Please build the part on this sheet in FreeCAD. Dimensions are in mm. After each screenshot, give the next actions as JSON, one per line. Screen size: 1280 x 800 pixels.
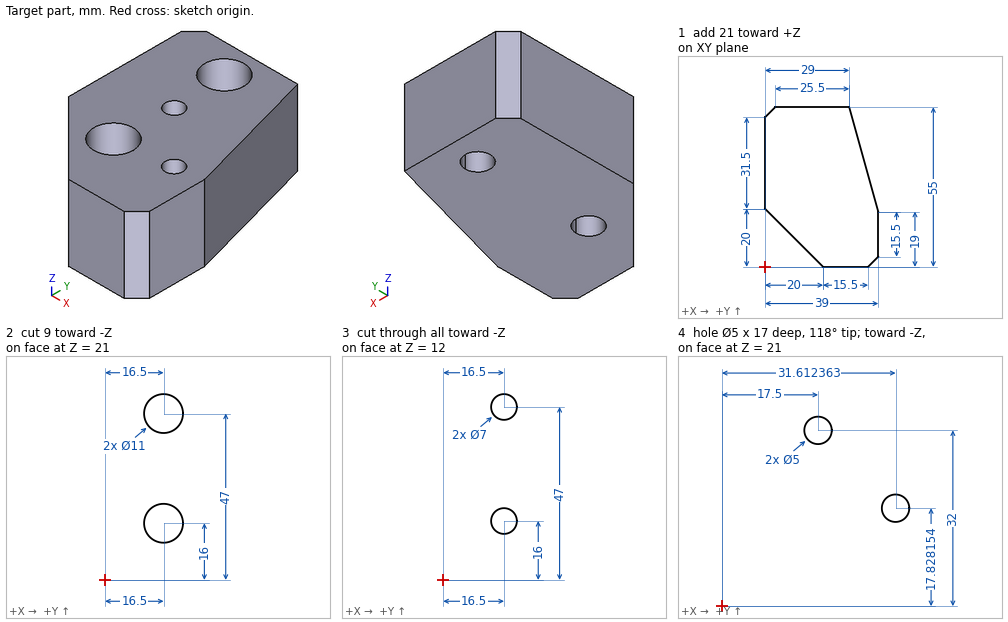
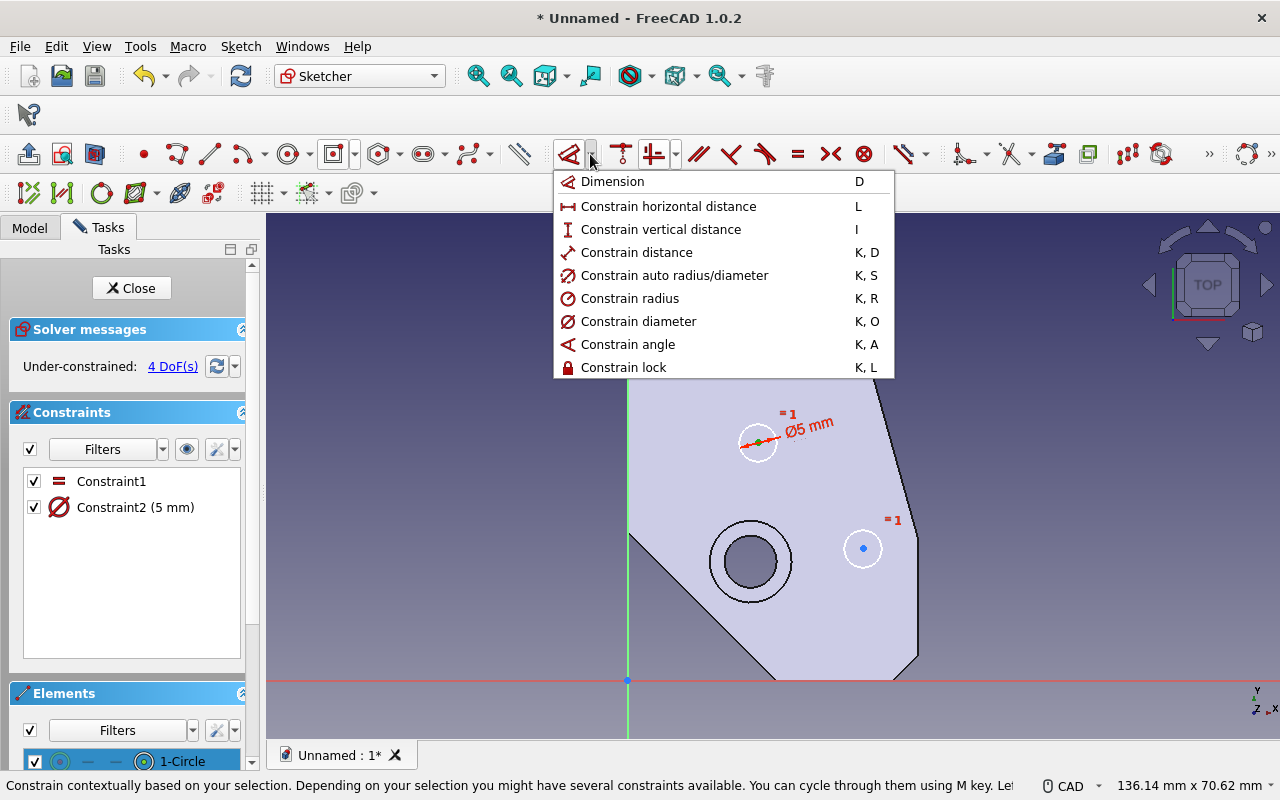
{"action": "left_click", "coordinate": [724, 230]}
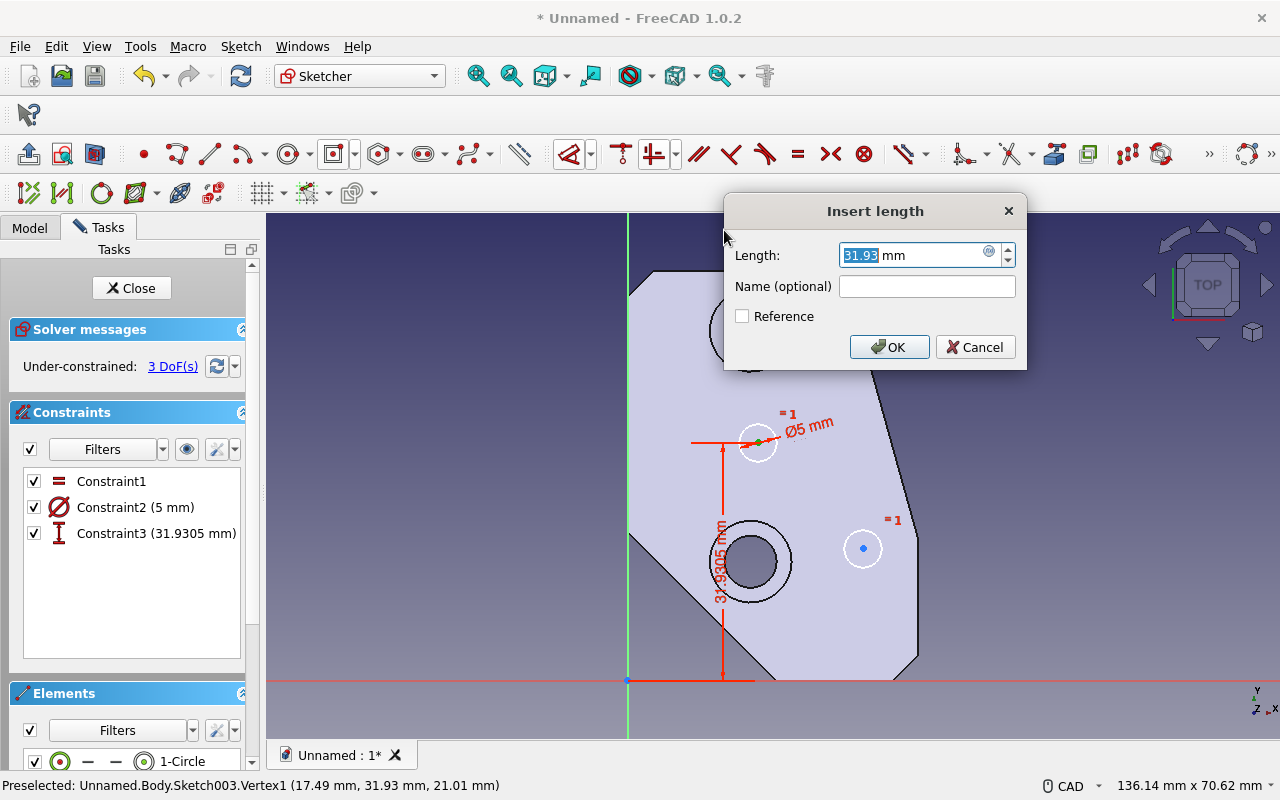
{"action": "type", "text": "32"}
{"action": "key", "text": "Return"}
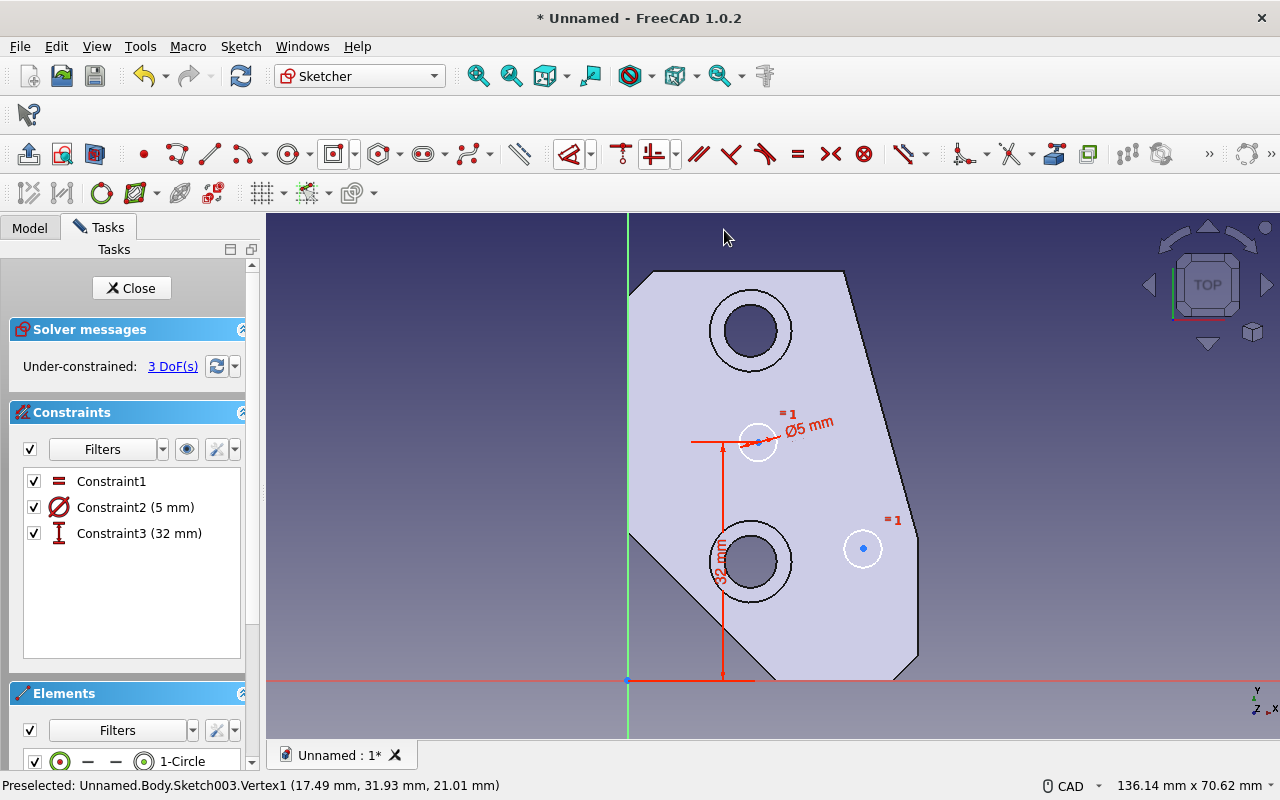
{"action": "left_click", "coordinate": [758, 442]}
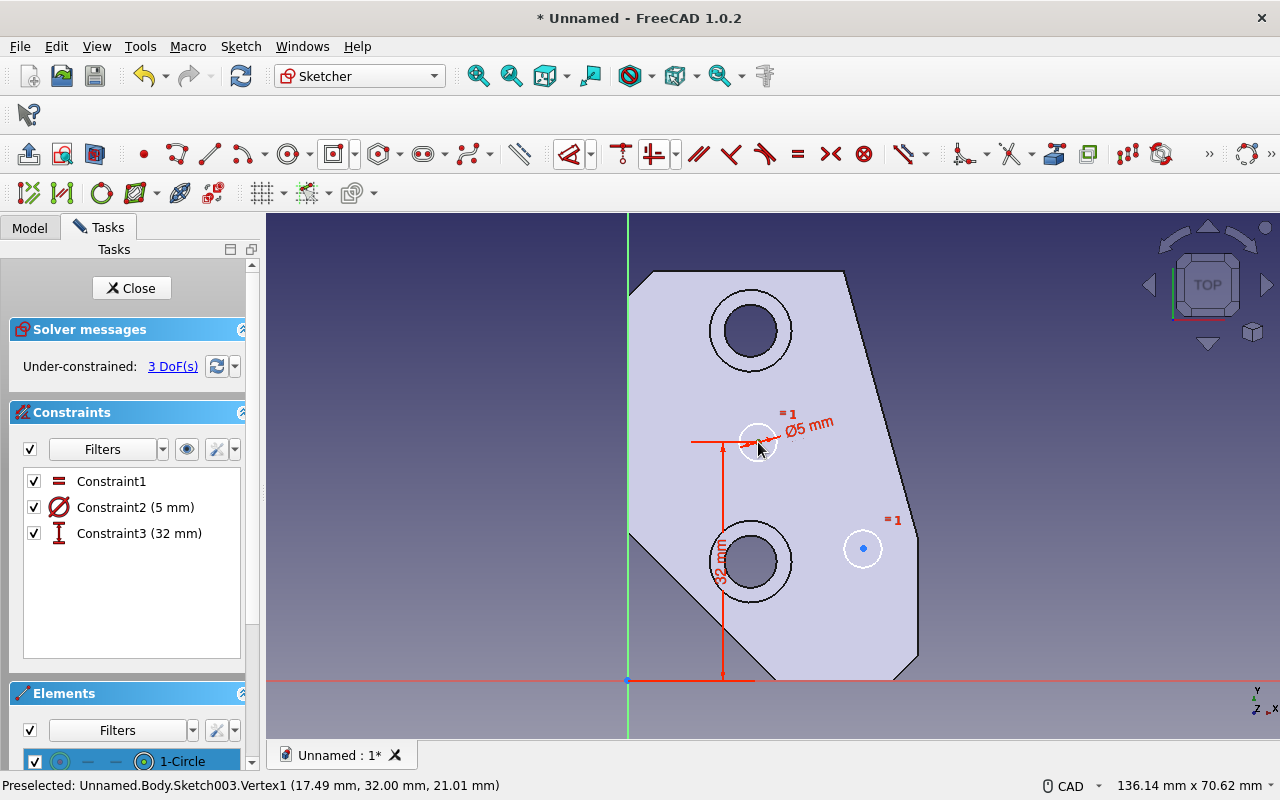
{"action": "key", "text": "l"}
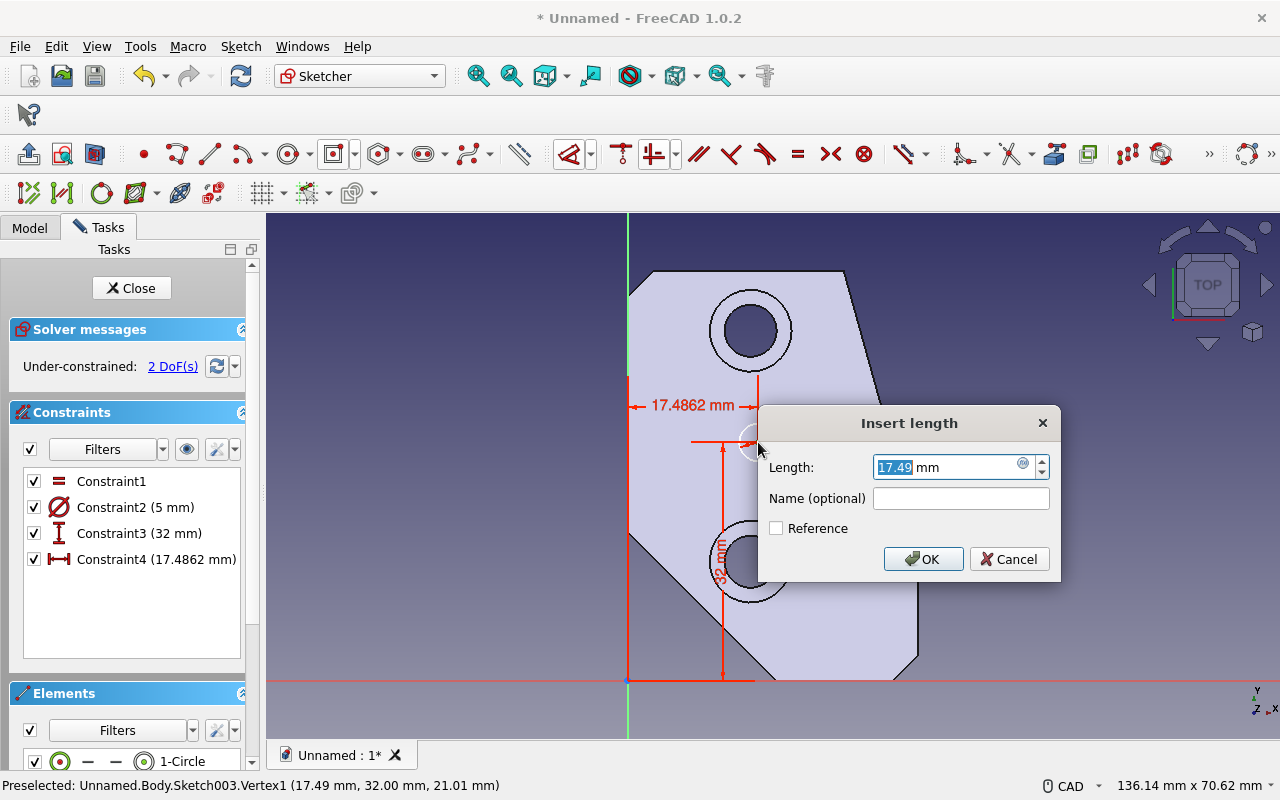
{"action": "type", "text": "17.5"}
{"action": "key", "text": "Return"}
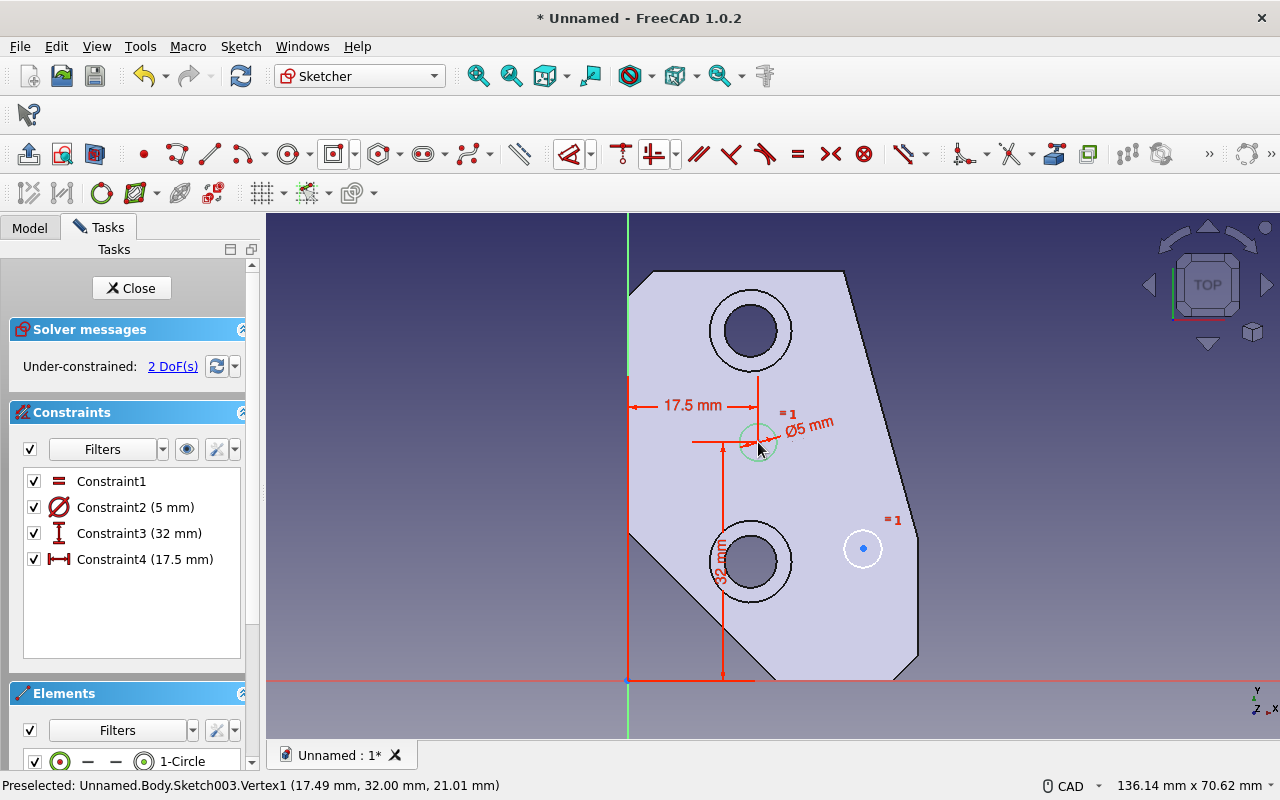
{"action": "left_click", "coordinate": [863, 549]}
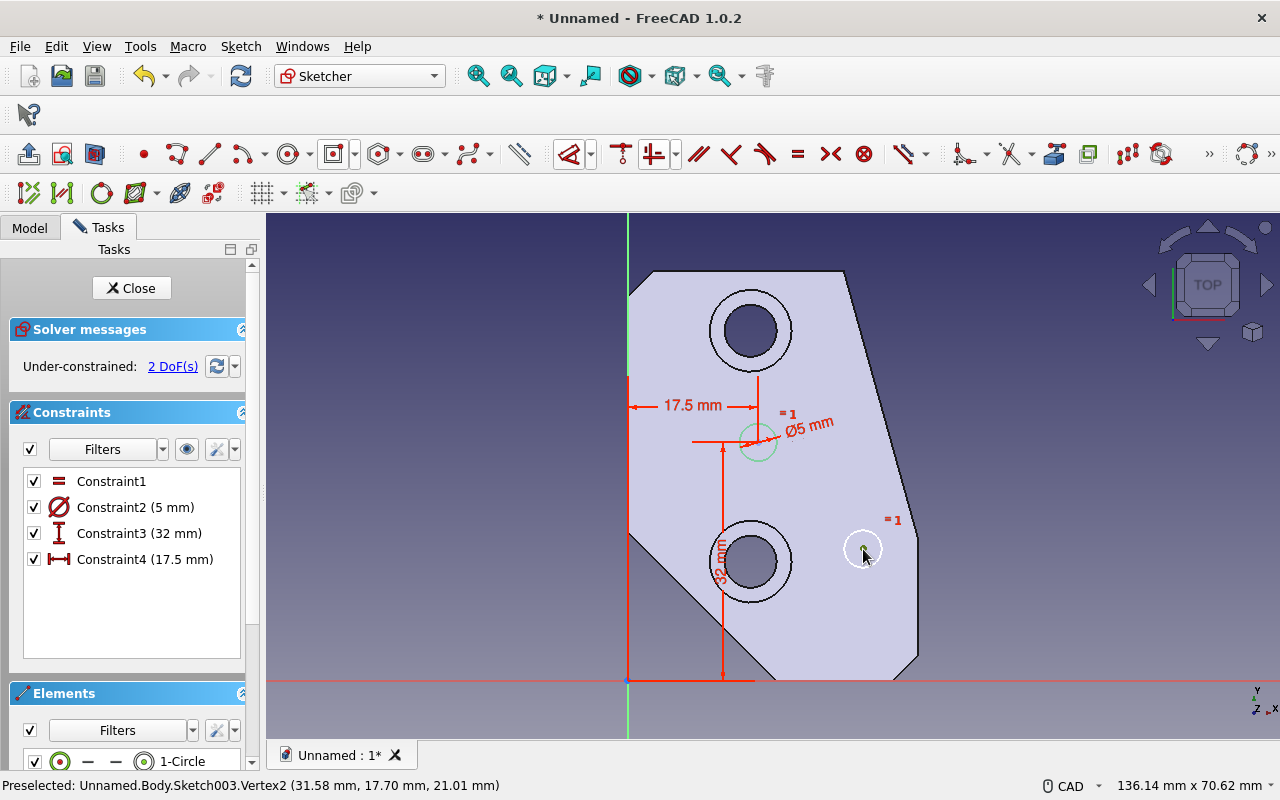
{"action": "left_click", "coordinate": [590, 154]}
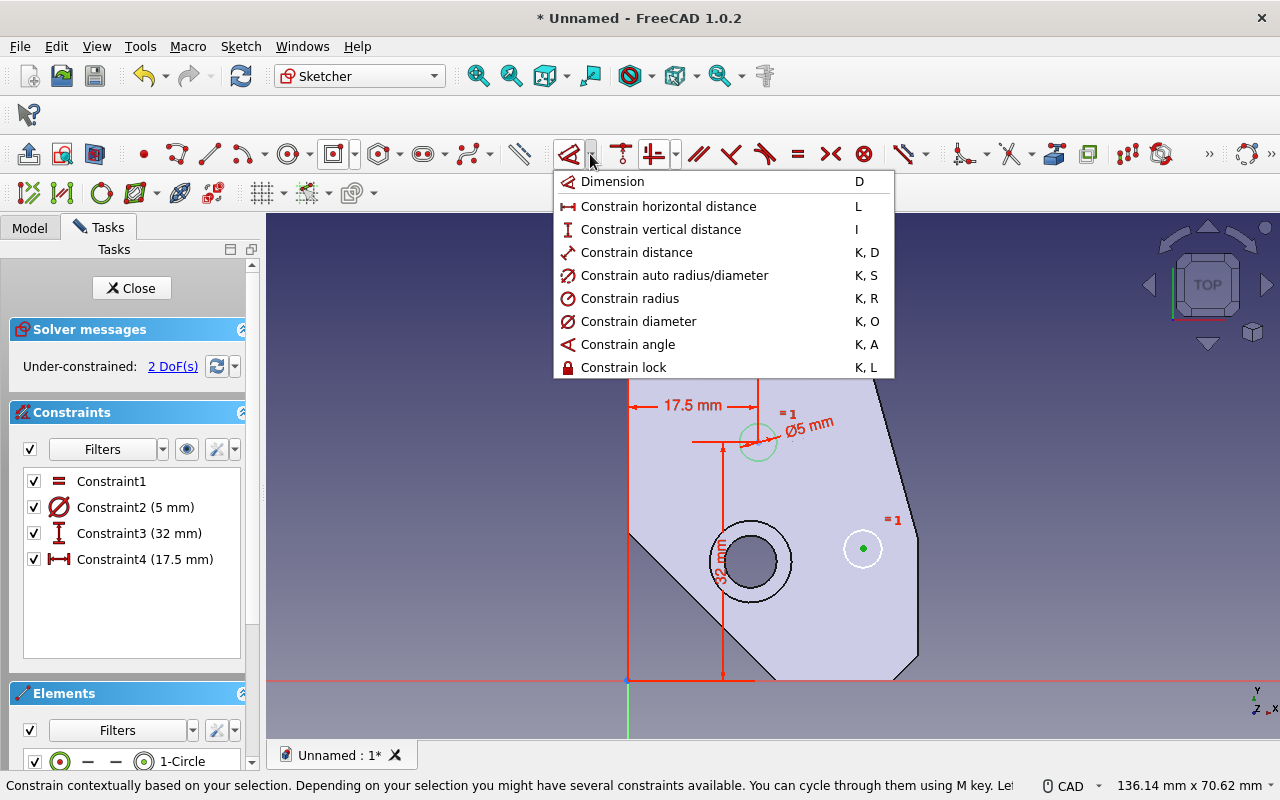
{"action": "left_click", "coordinate": [724, 206]}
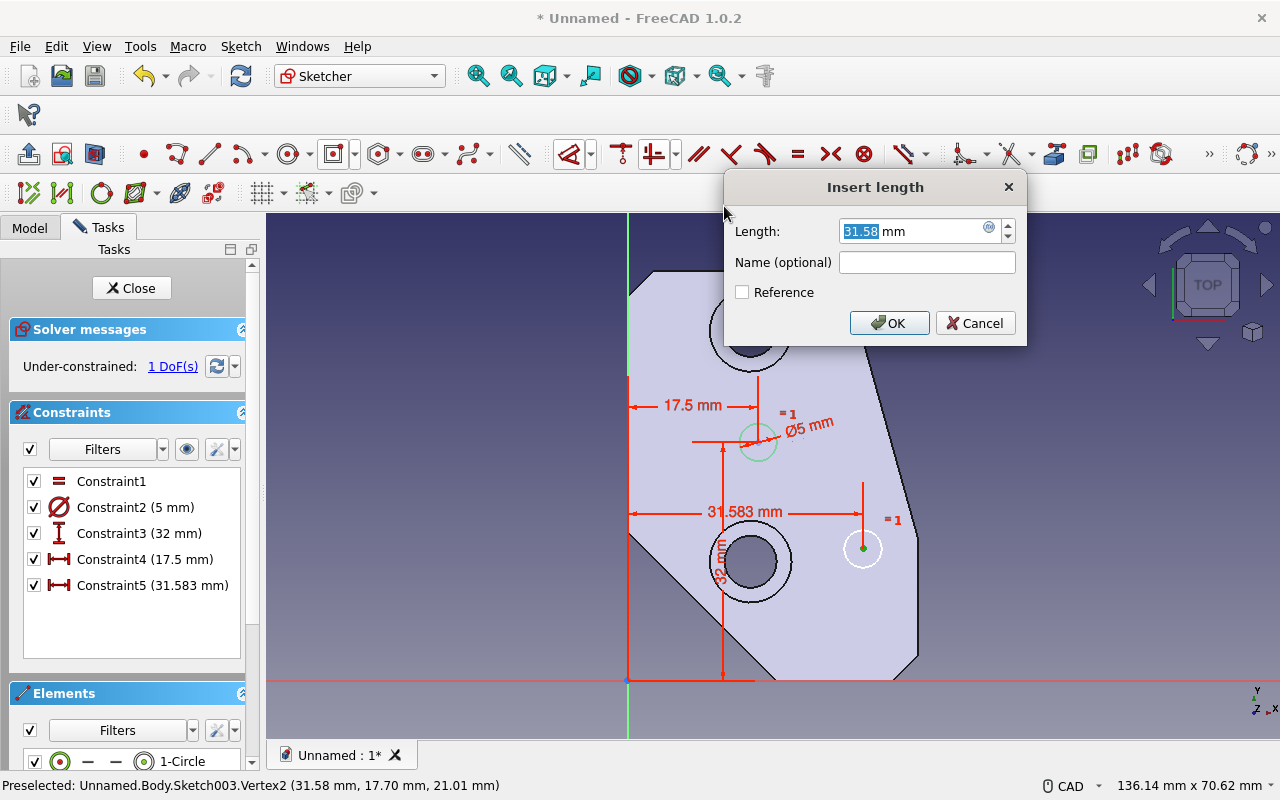
{"action": "type", "text": "31.612363"}
{"action": "key", "text": "Return"}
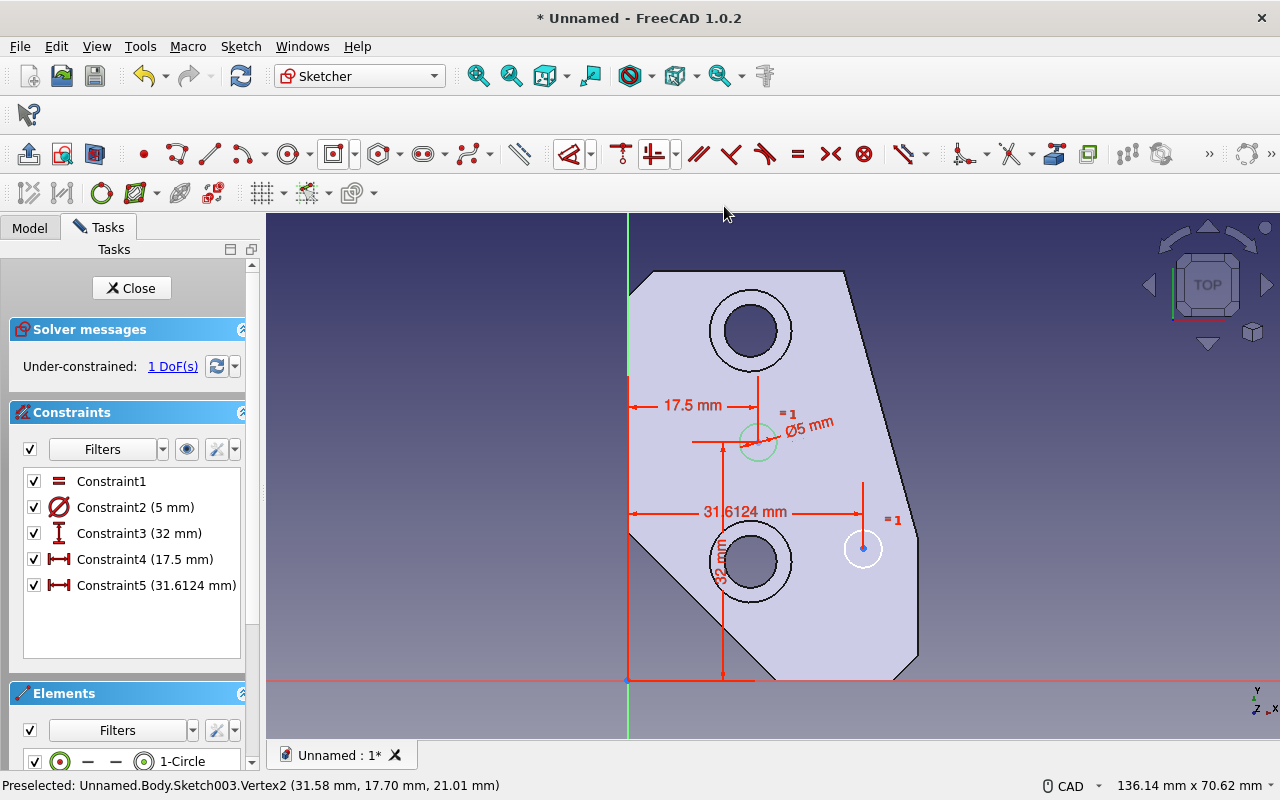
{"action": "left_click", "coordinate": [863, 549]}